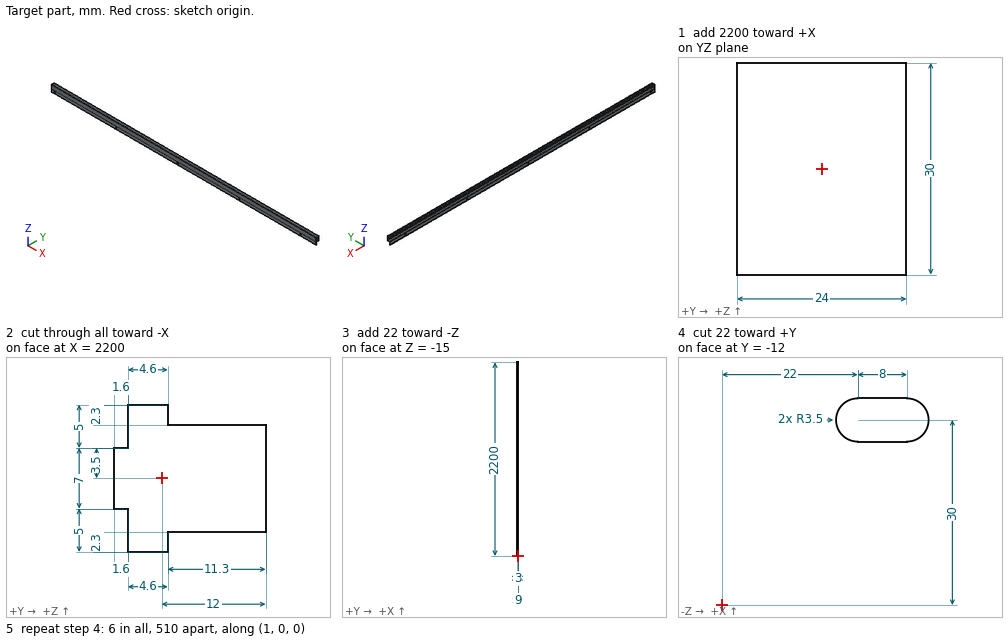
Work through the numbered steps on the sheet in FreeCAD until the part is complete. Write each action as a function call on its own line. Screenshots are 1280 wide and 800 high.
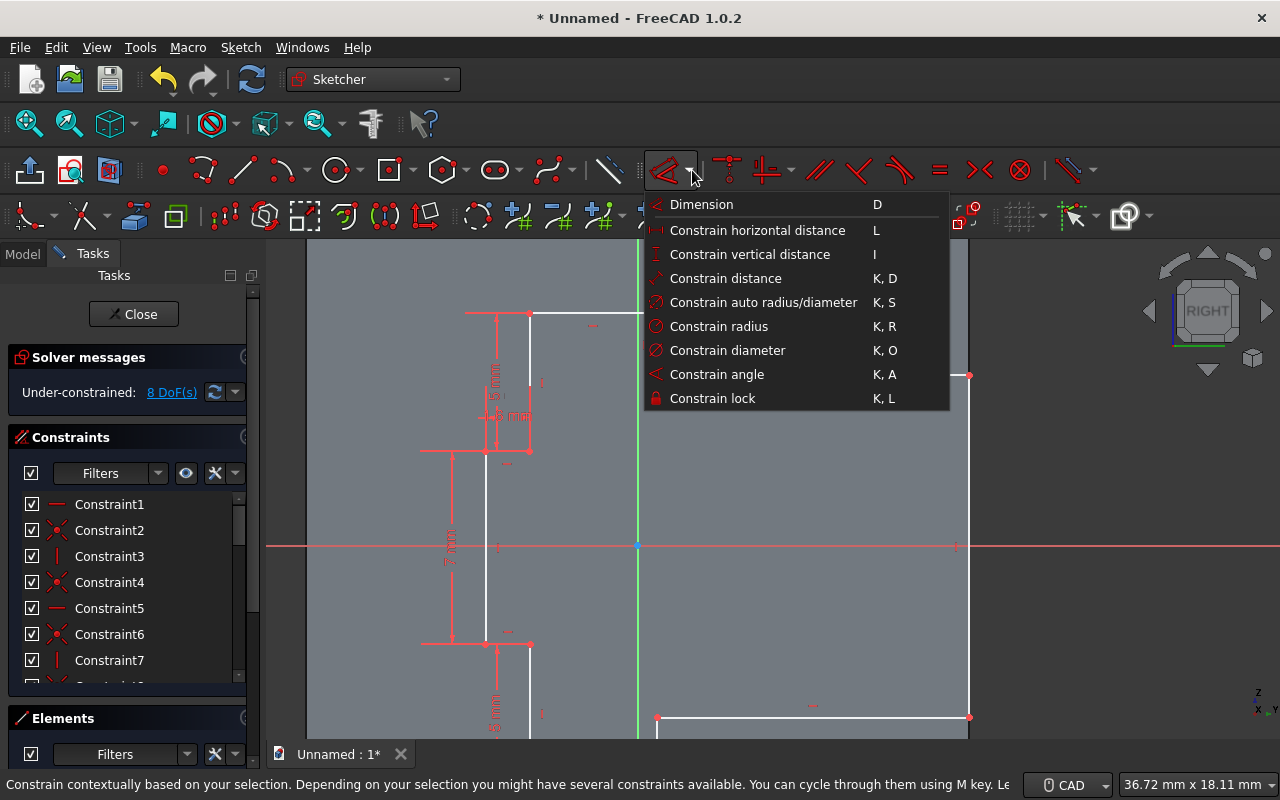
click(797, 230)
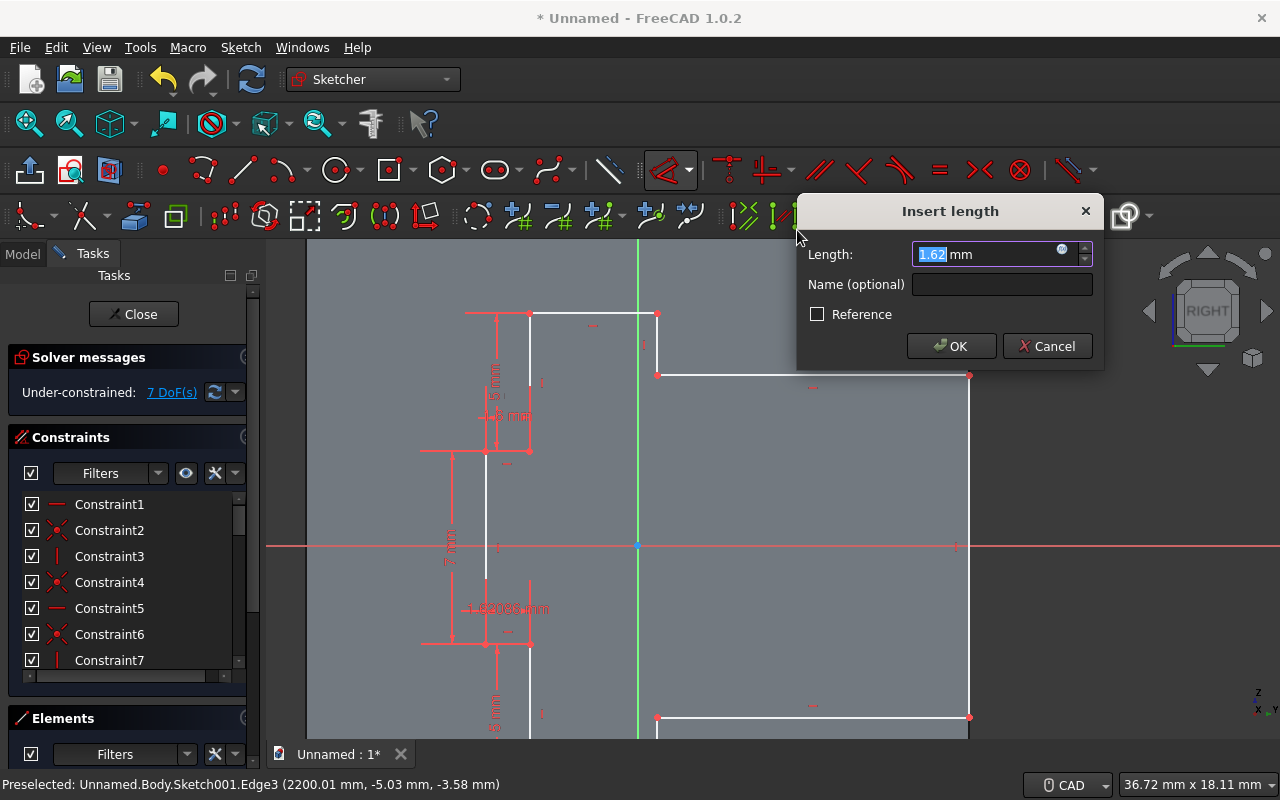
text(1.6)
key(Return)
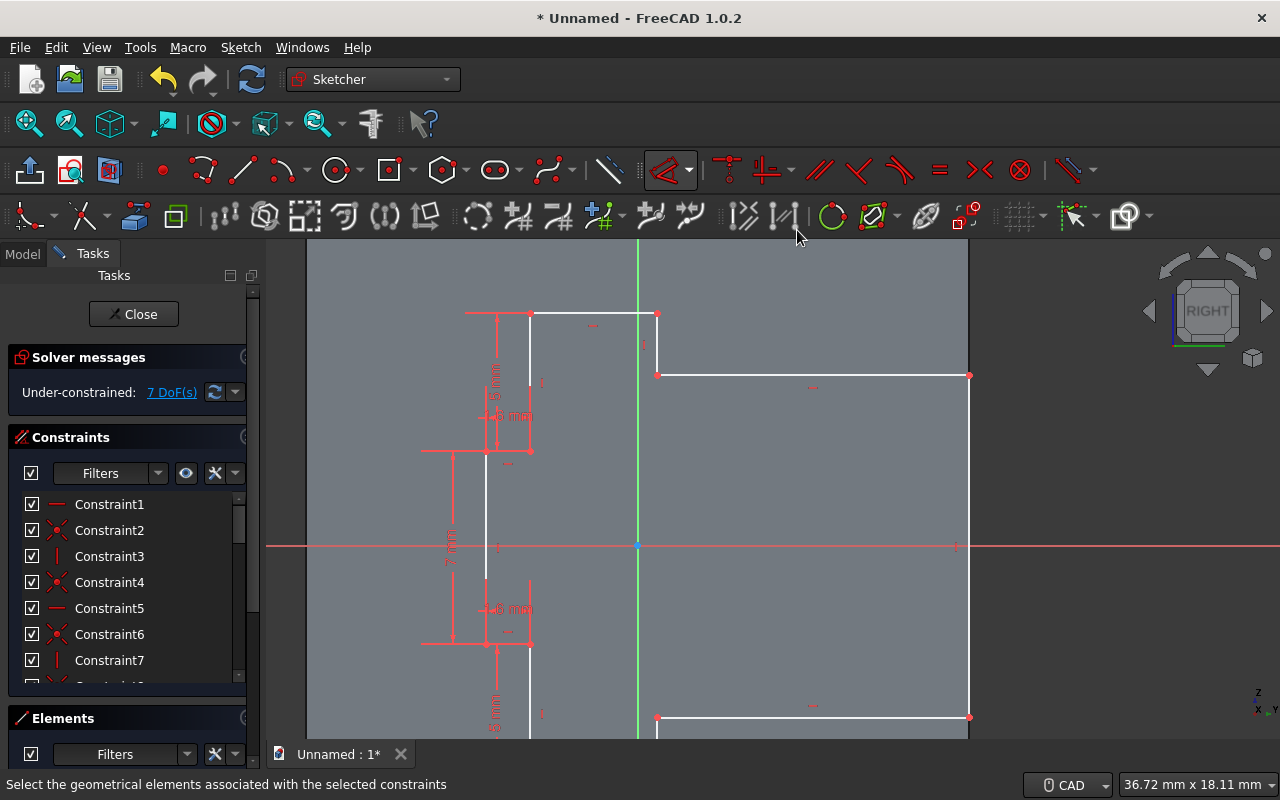
scroll(658, 374, down, 2)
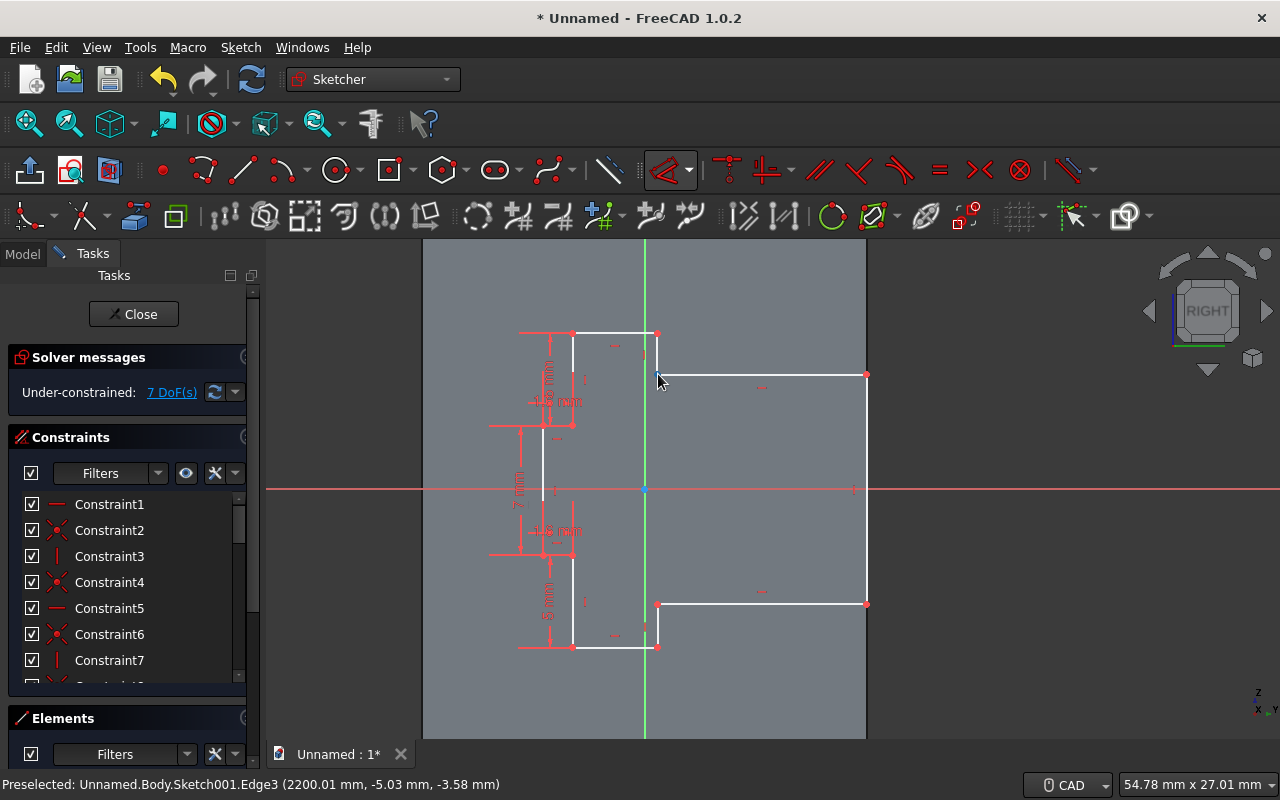
click(598, 648)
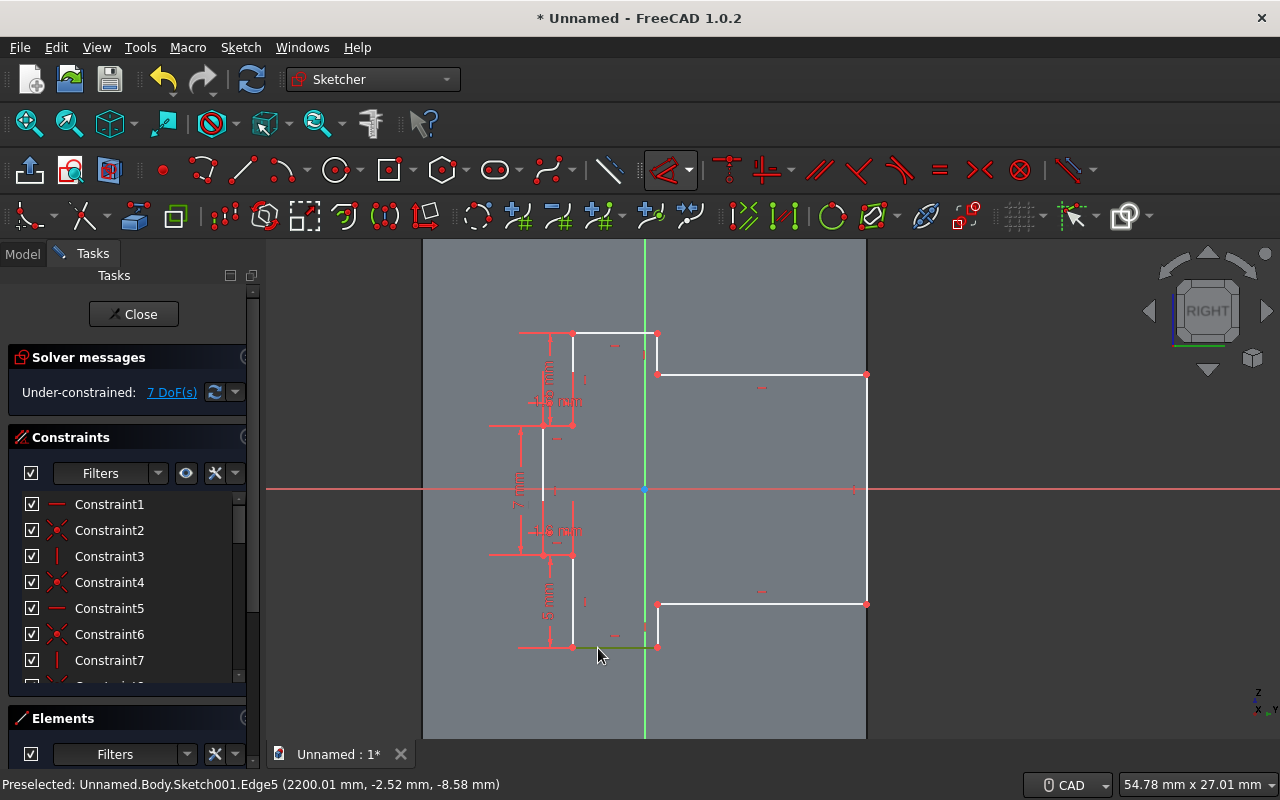
key(l)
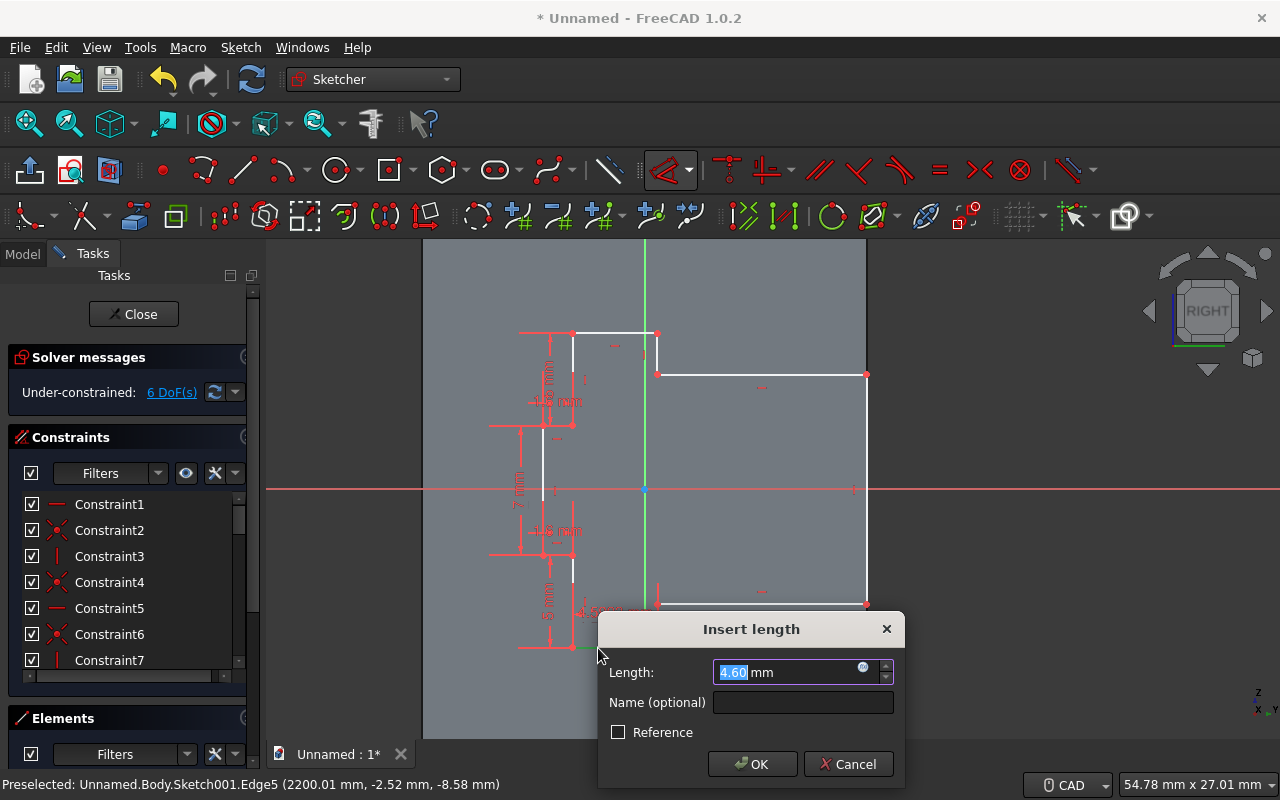
text(4.6)
key(Return)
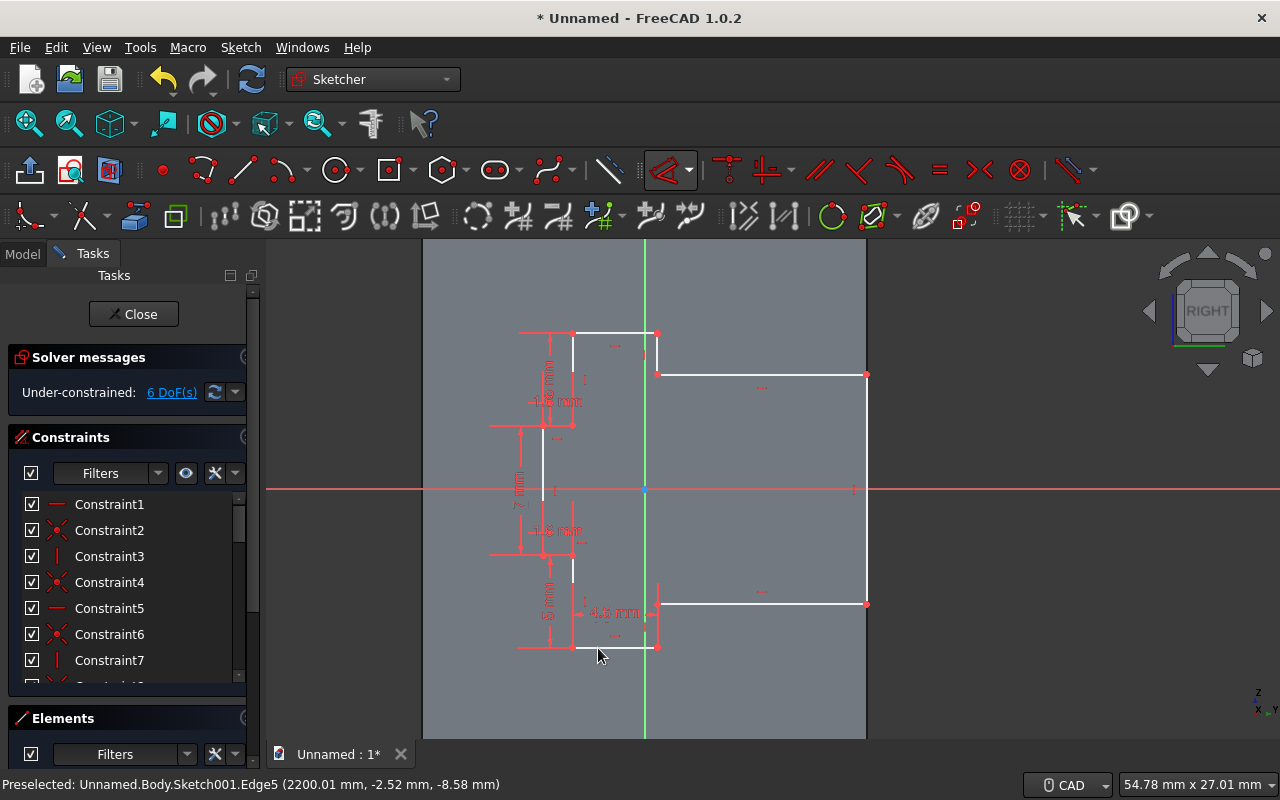
click(658, 635)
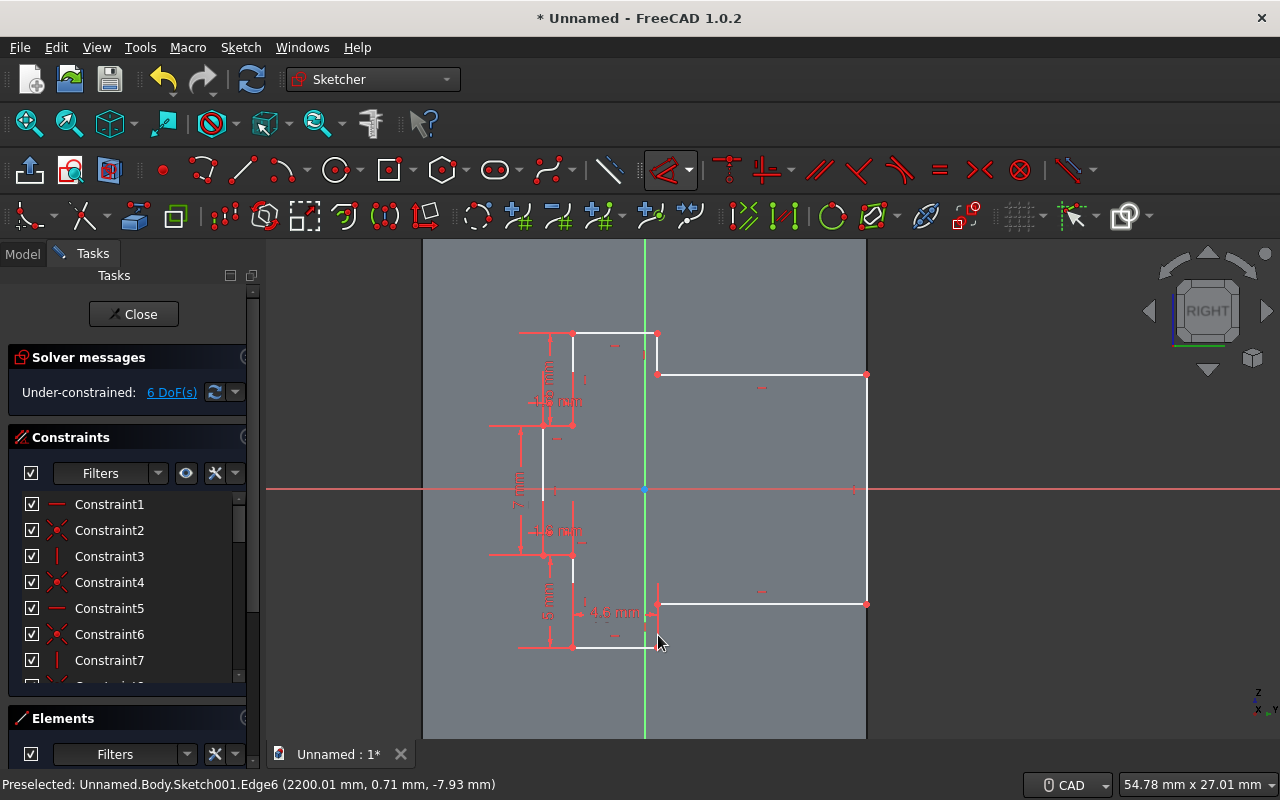
click(692, 170)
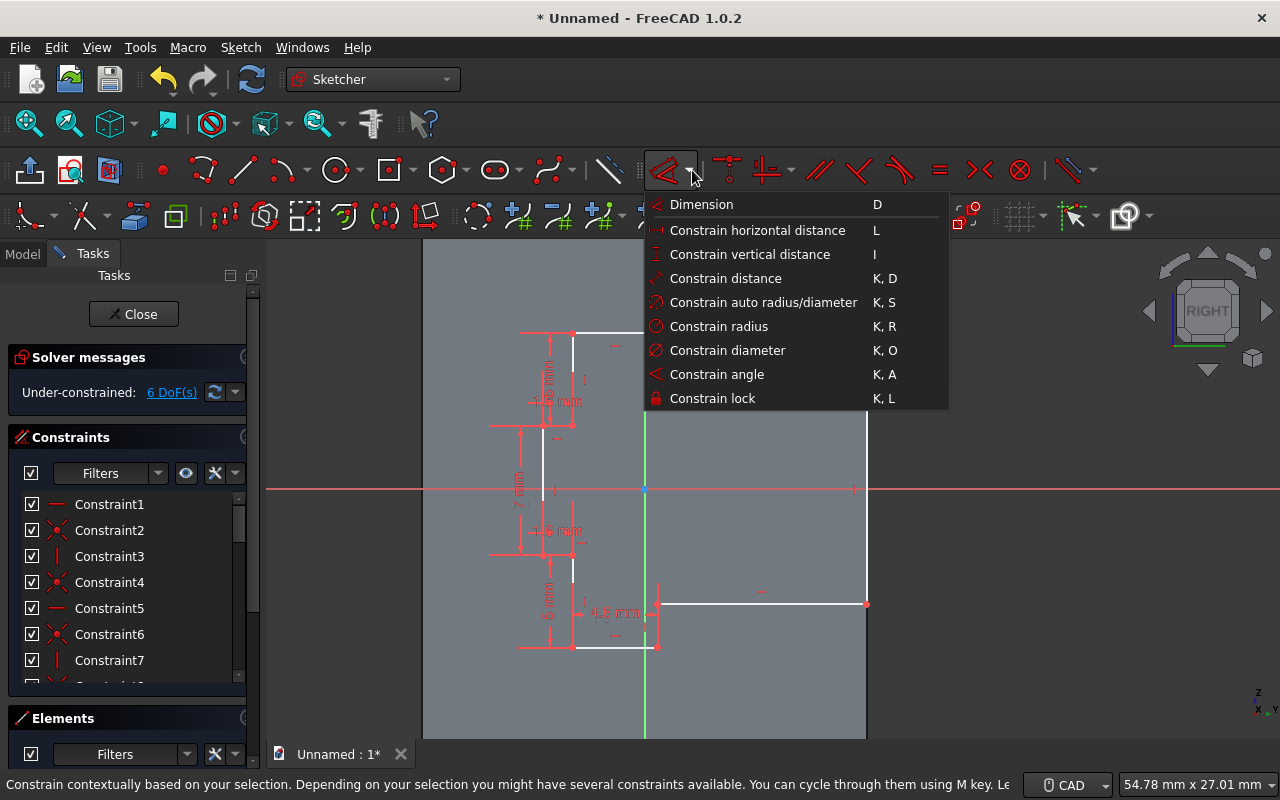
click(797, 254)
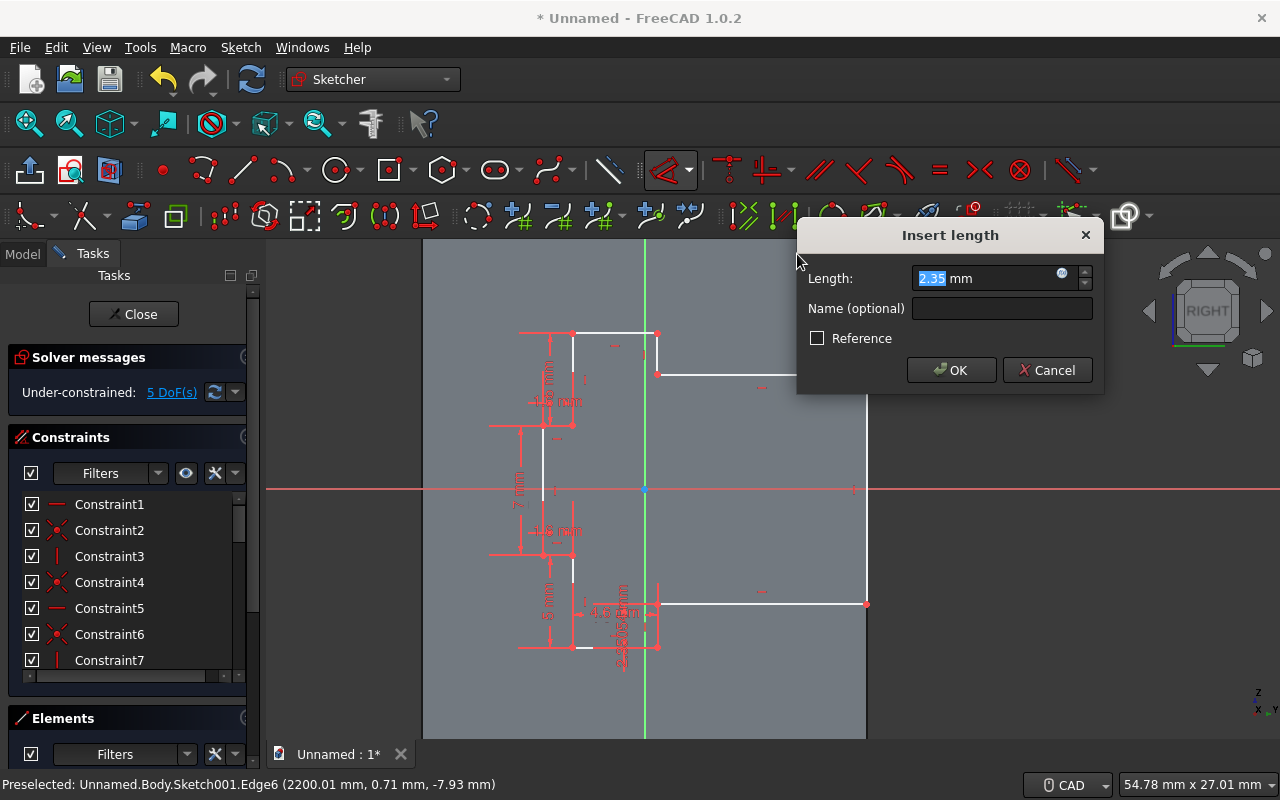
text(2.3)
key(Return)